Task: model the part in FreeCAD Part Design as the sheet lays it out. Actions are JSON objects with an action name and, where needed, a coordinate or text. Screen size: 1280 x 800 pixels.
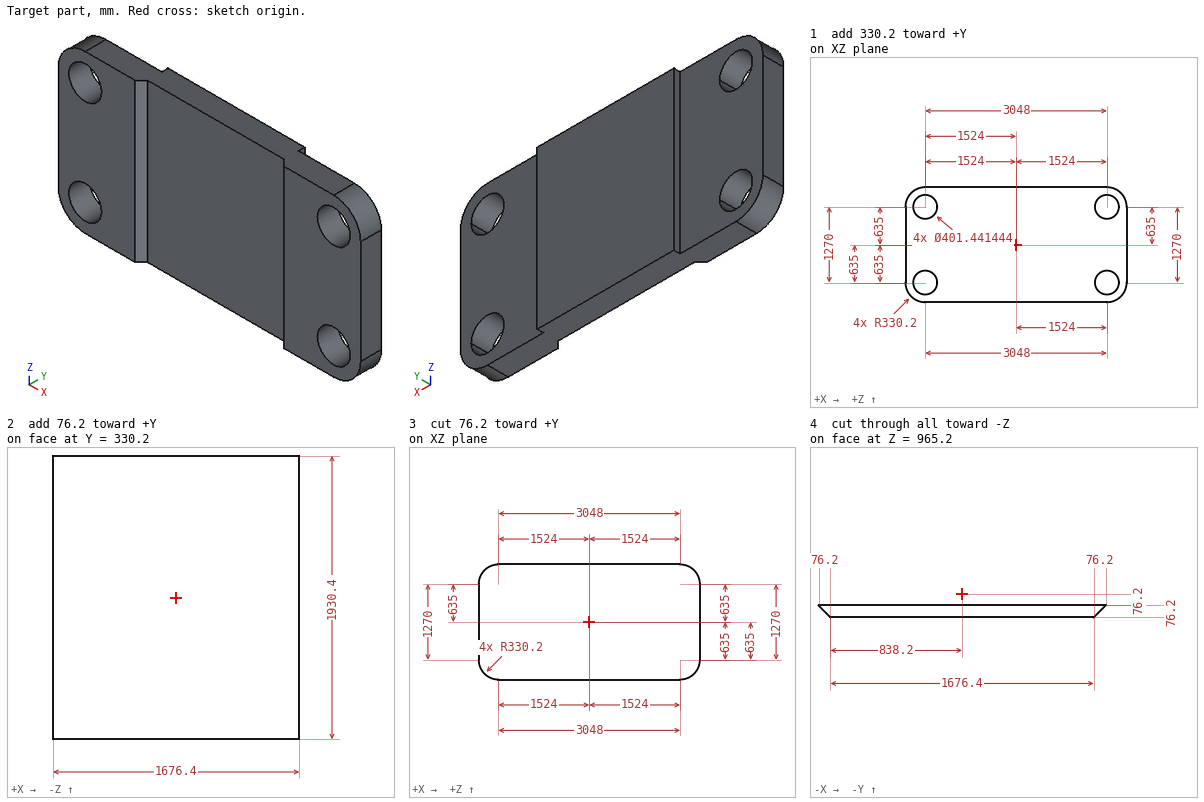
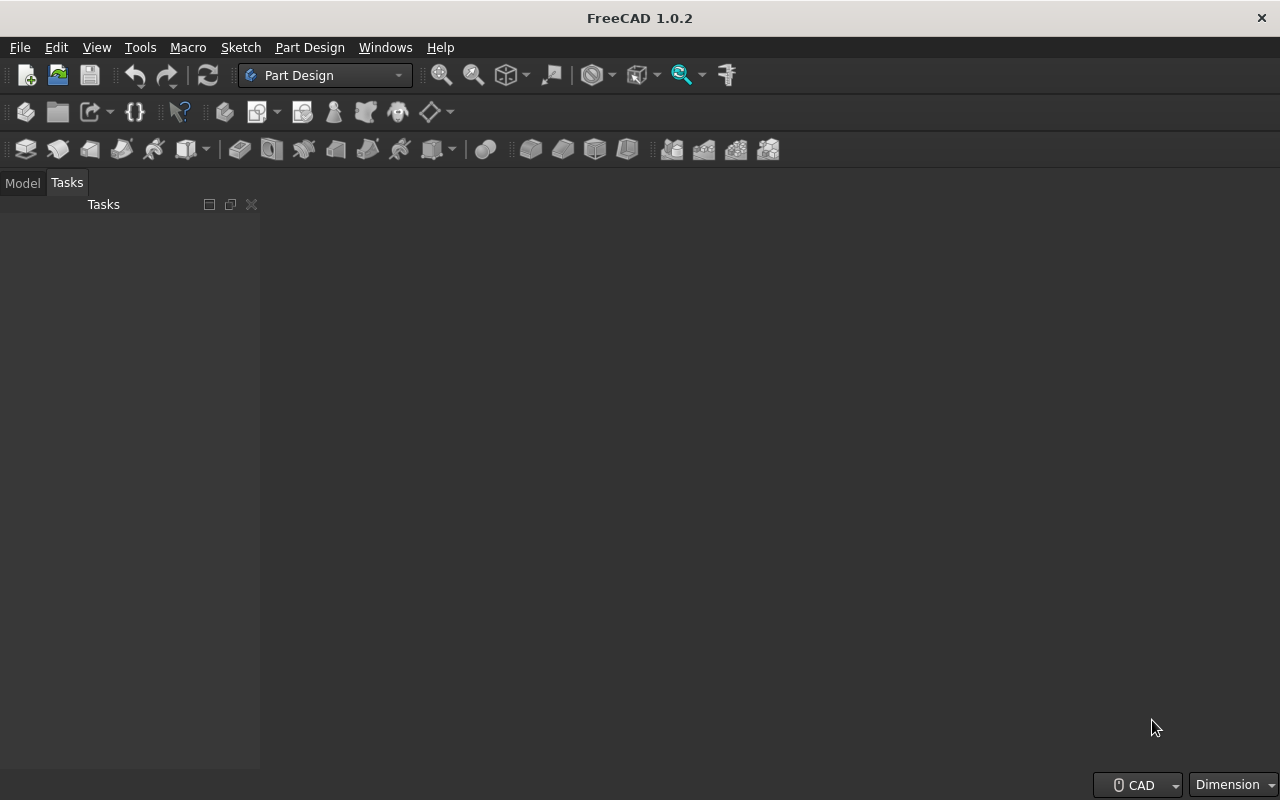
{"action": "key", "text": "ctrl+n"}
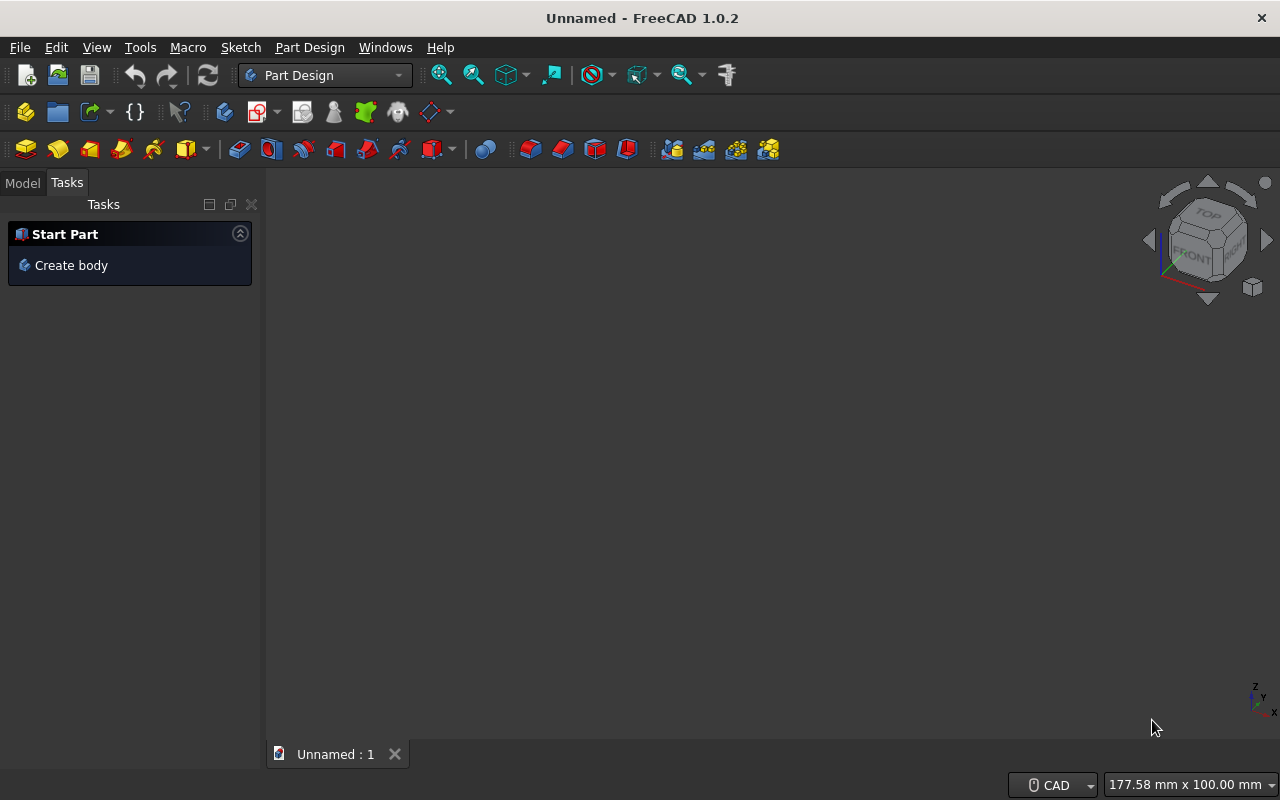
{"action": "left_click", "coordinate": [258, 112]}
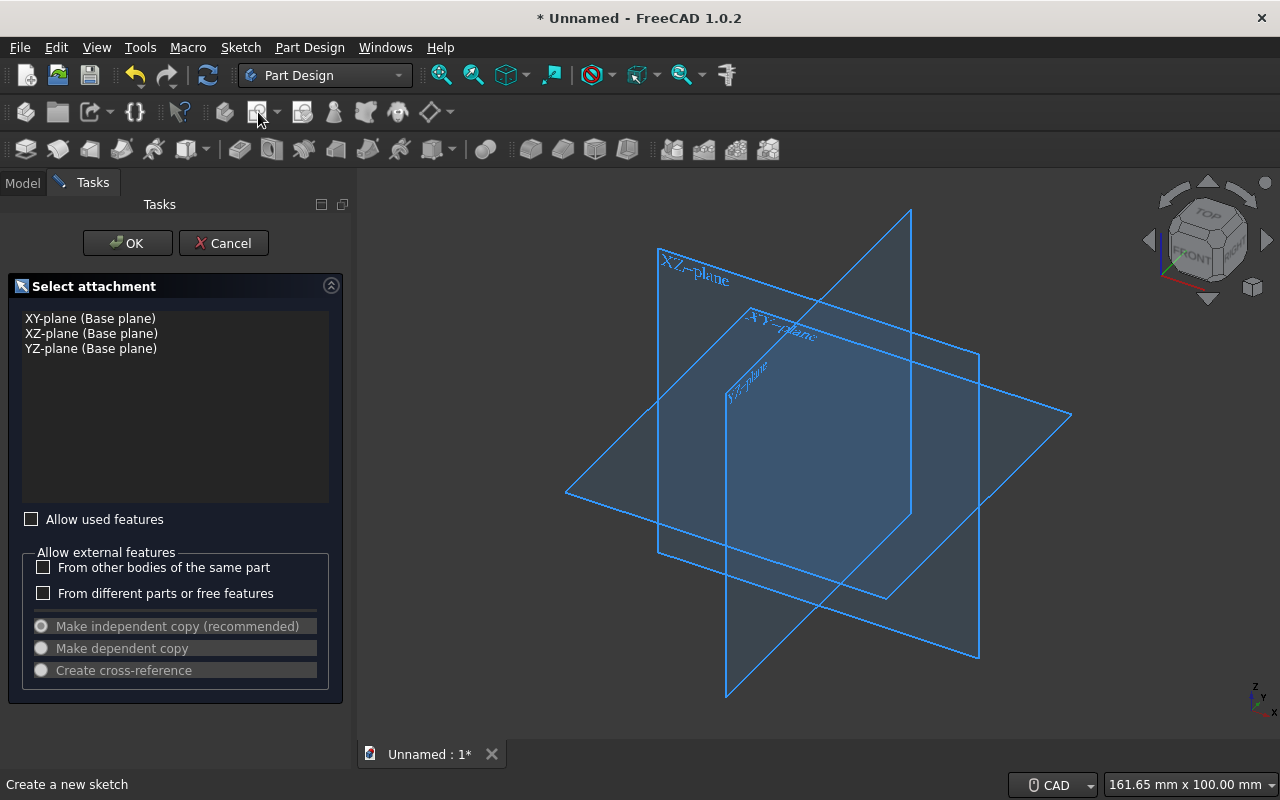
{"action": "left_click", "coordinate": [82, 334]}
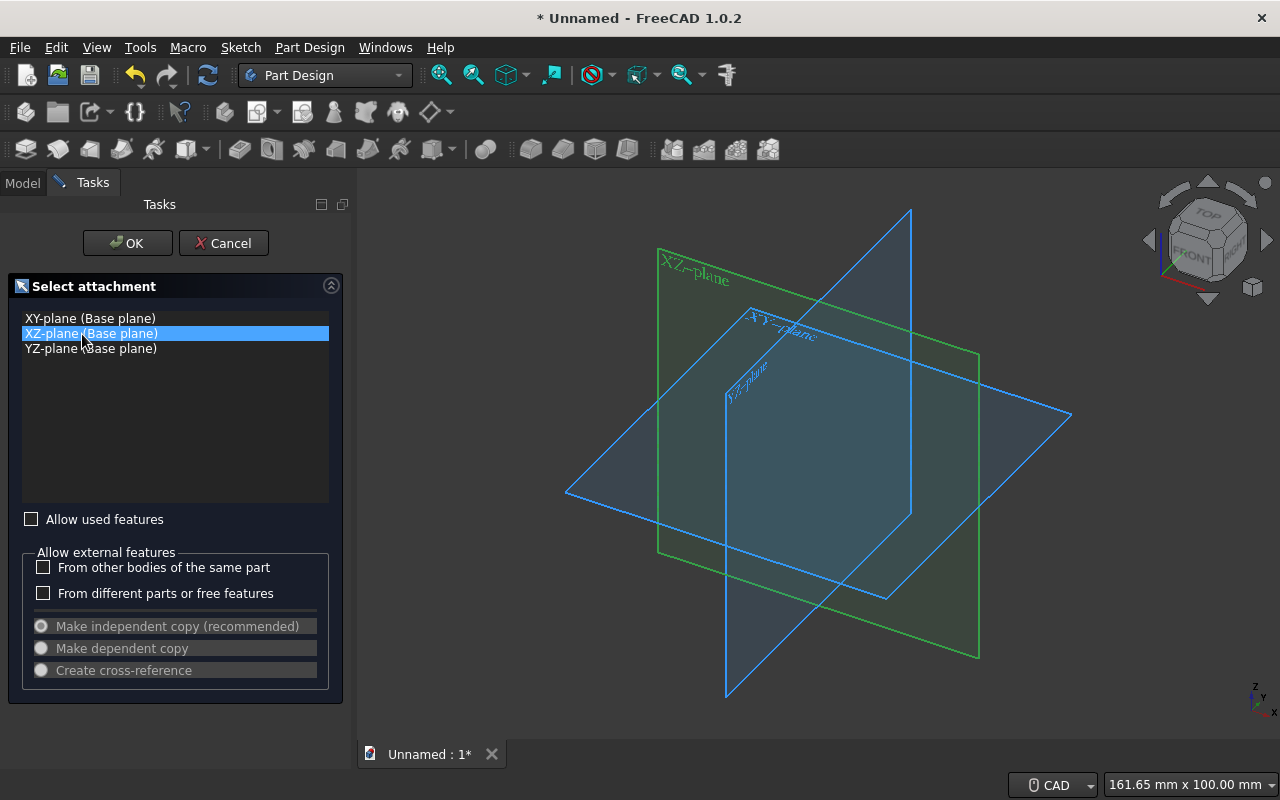
{"action": "left_click", "coordinate": [128, 243]}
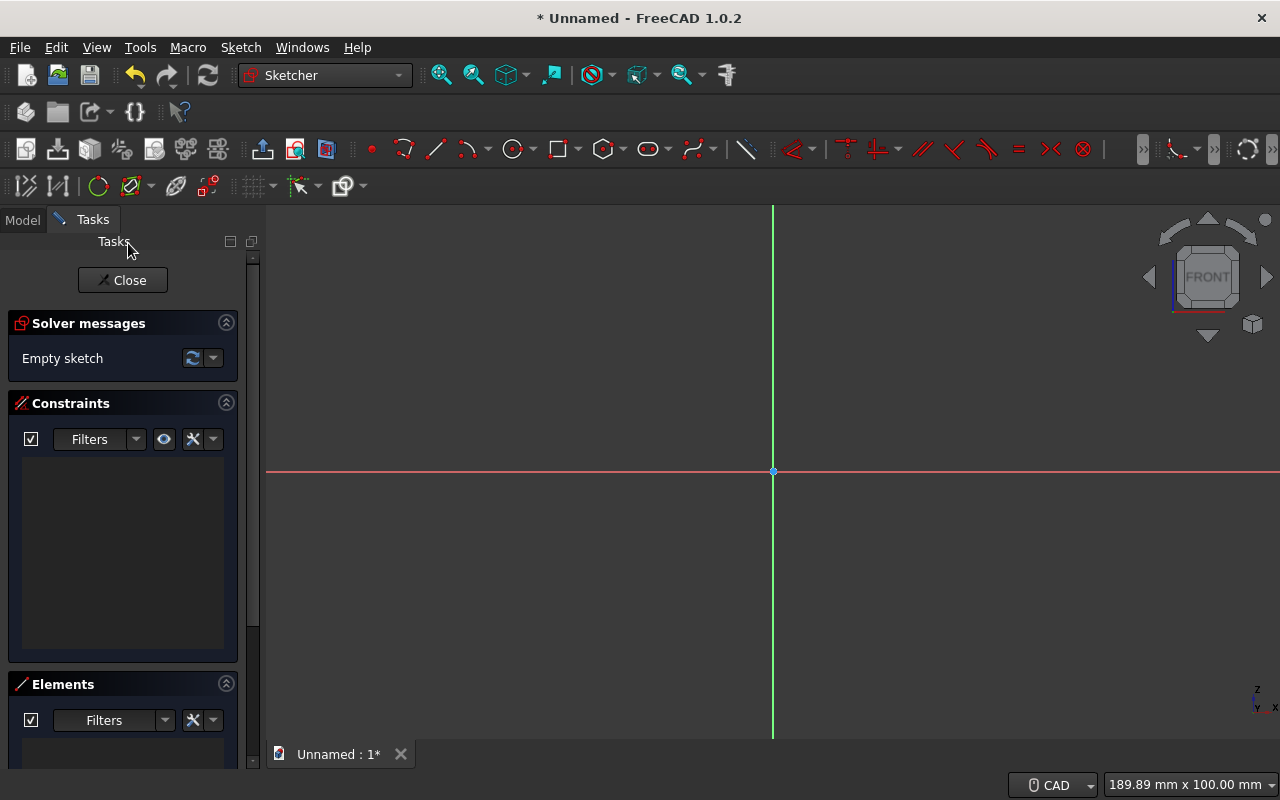
{"action": "scroll", "coordinate": [702, 472], "scroll_direction": "down", "scroll_amount": 17}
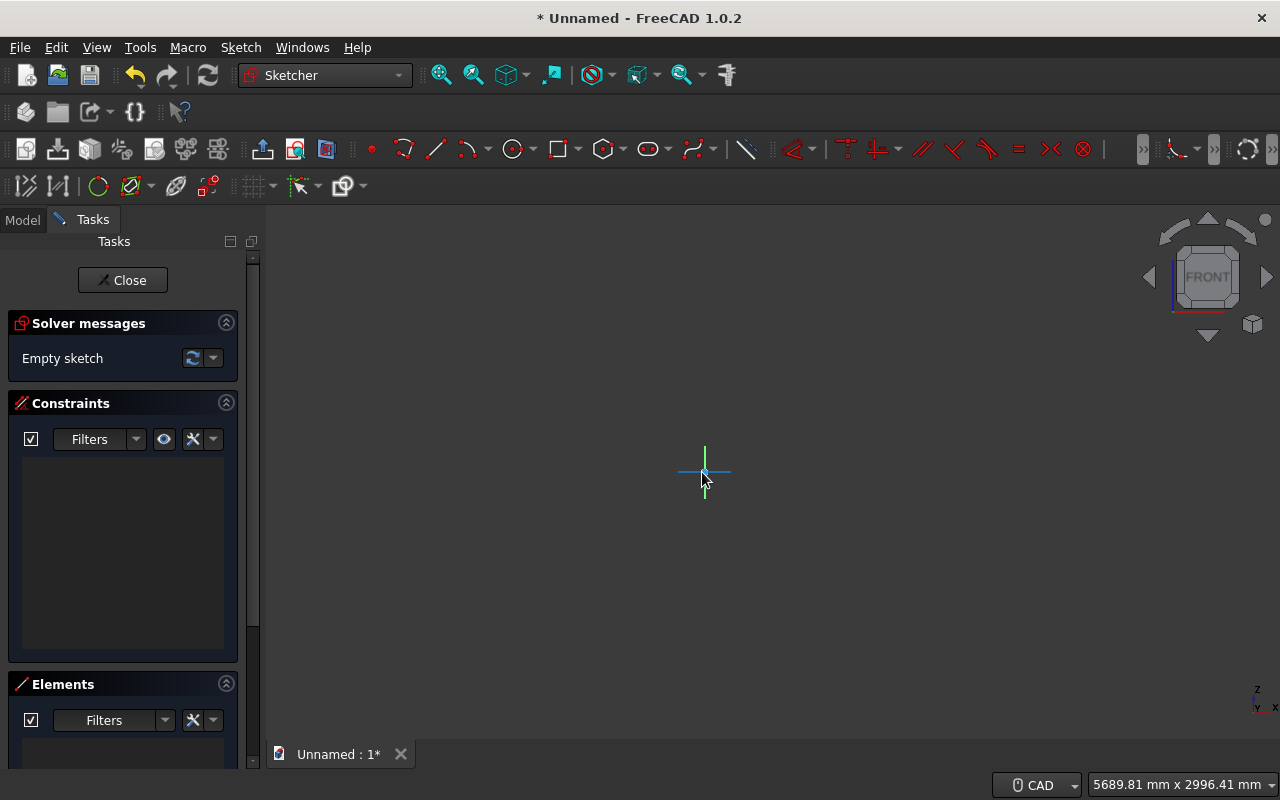
{"action": "key", "text": "g l"}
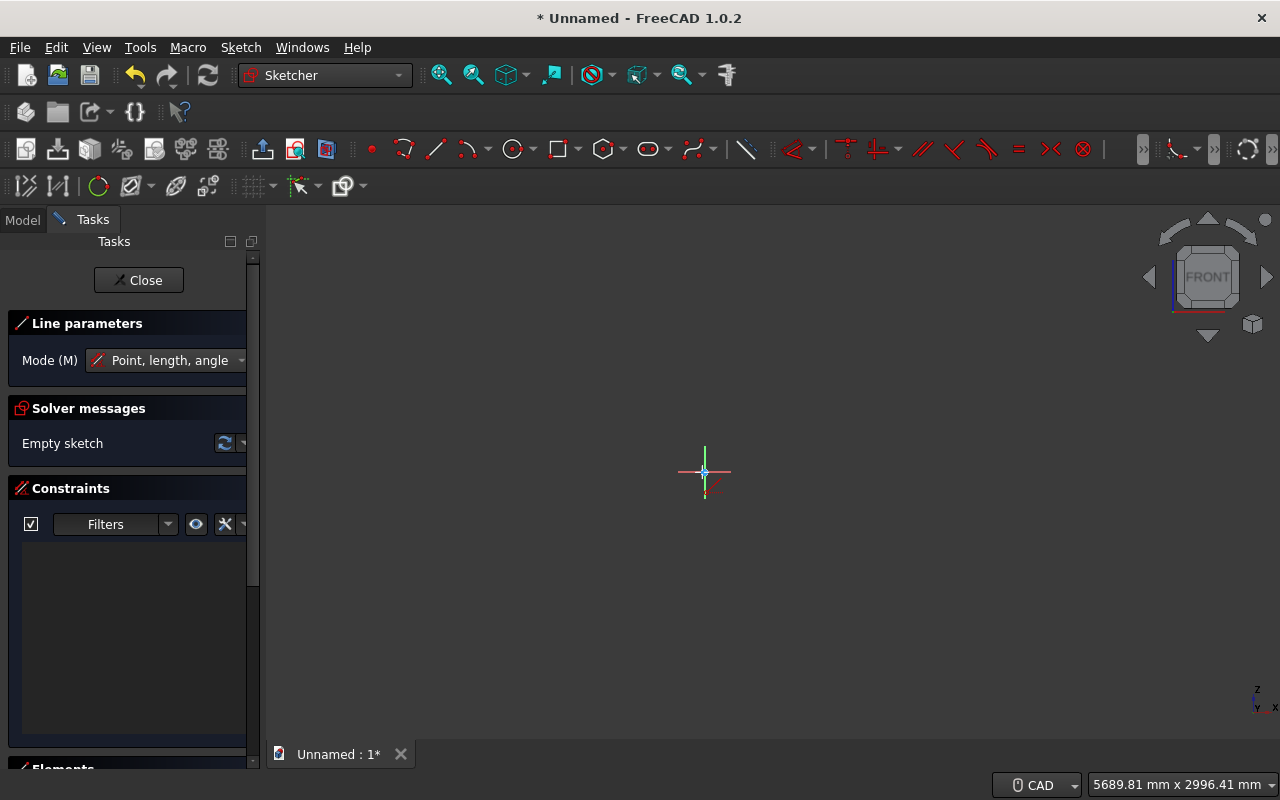
{"action": "left_click", "coordinate": [976, 644]}
{"action": "left_click", "coordinate": [433, 644]}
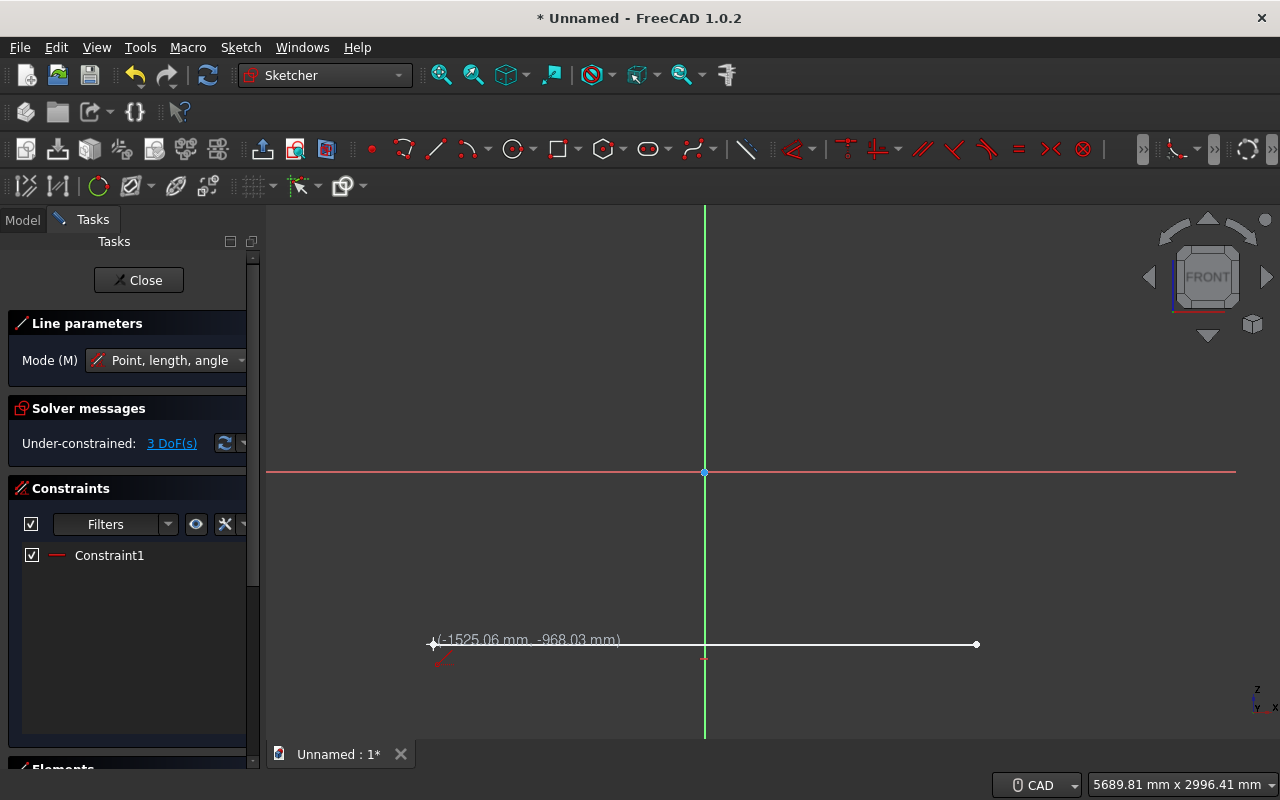
{"action": "left_click", "coordinate": [374, 586]}
{"action": "left_click", "coordinate": [374, 359]}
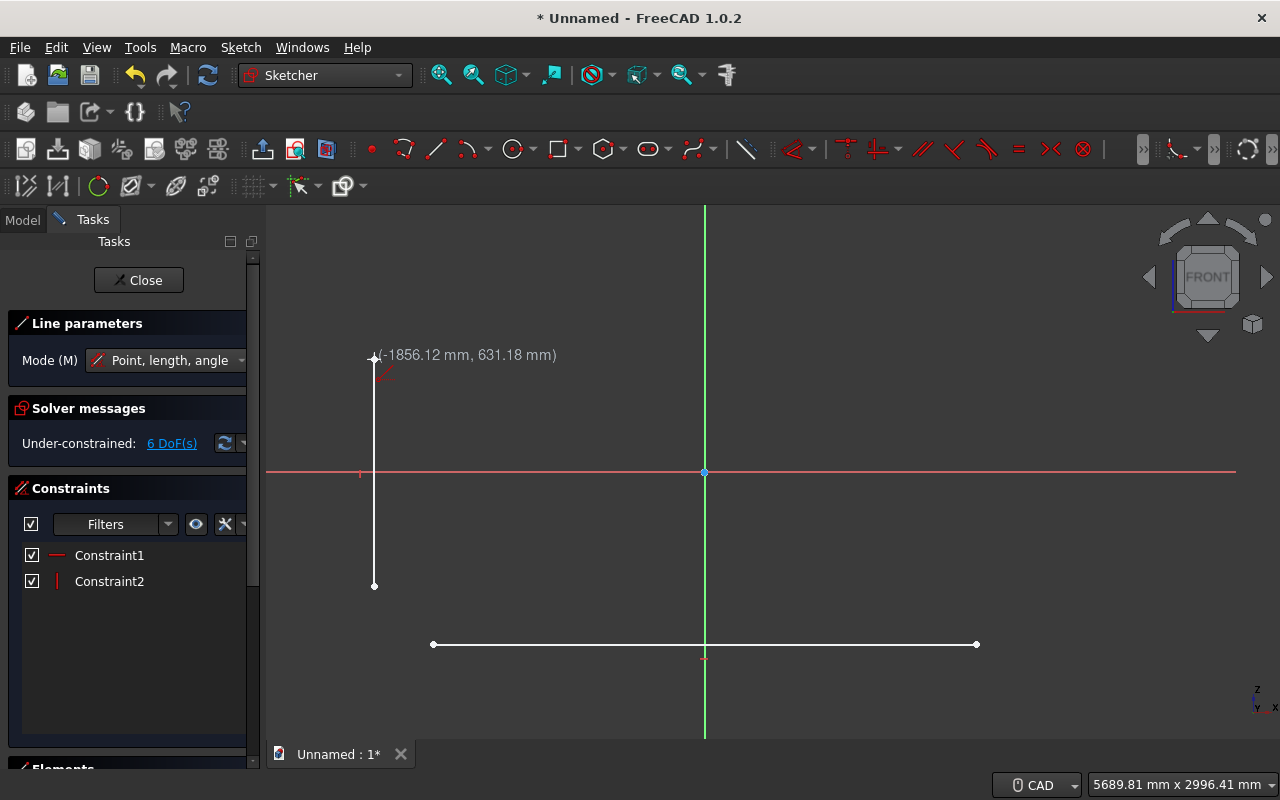
{"action": "left_click", "coordinate": [433, 300]}
{"action": "left_click", "coordinate": [976, 300]}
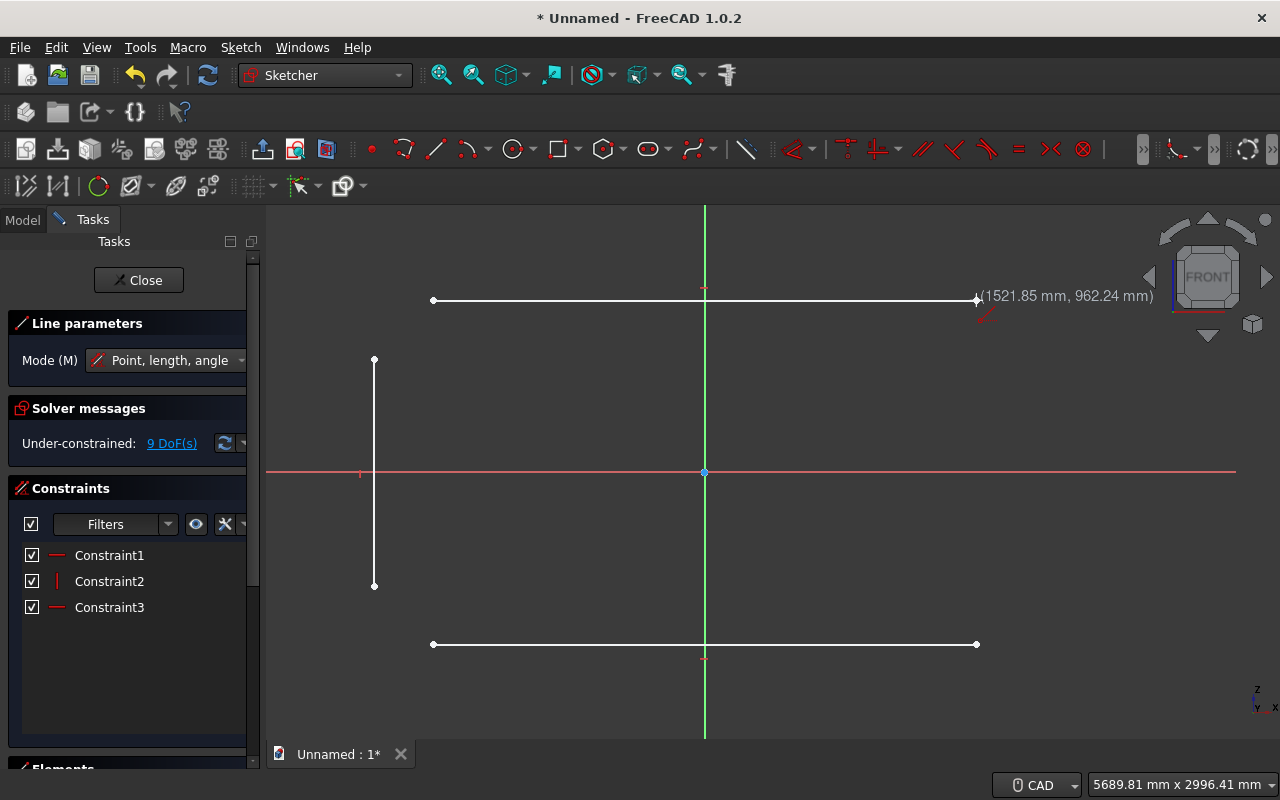
{"action": "left_click", "coordinate": [1035, 359]}
{"action": "left_click", "coordinate": [1035, 586]}